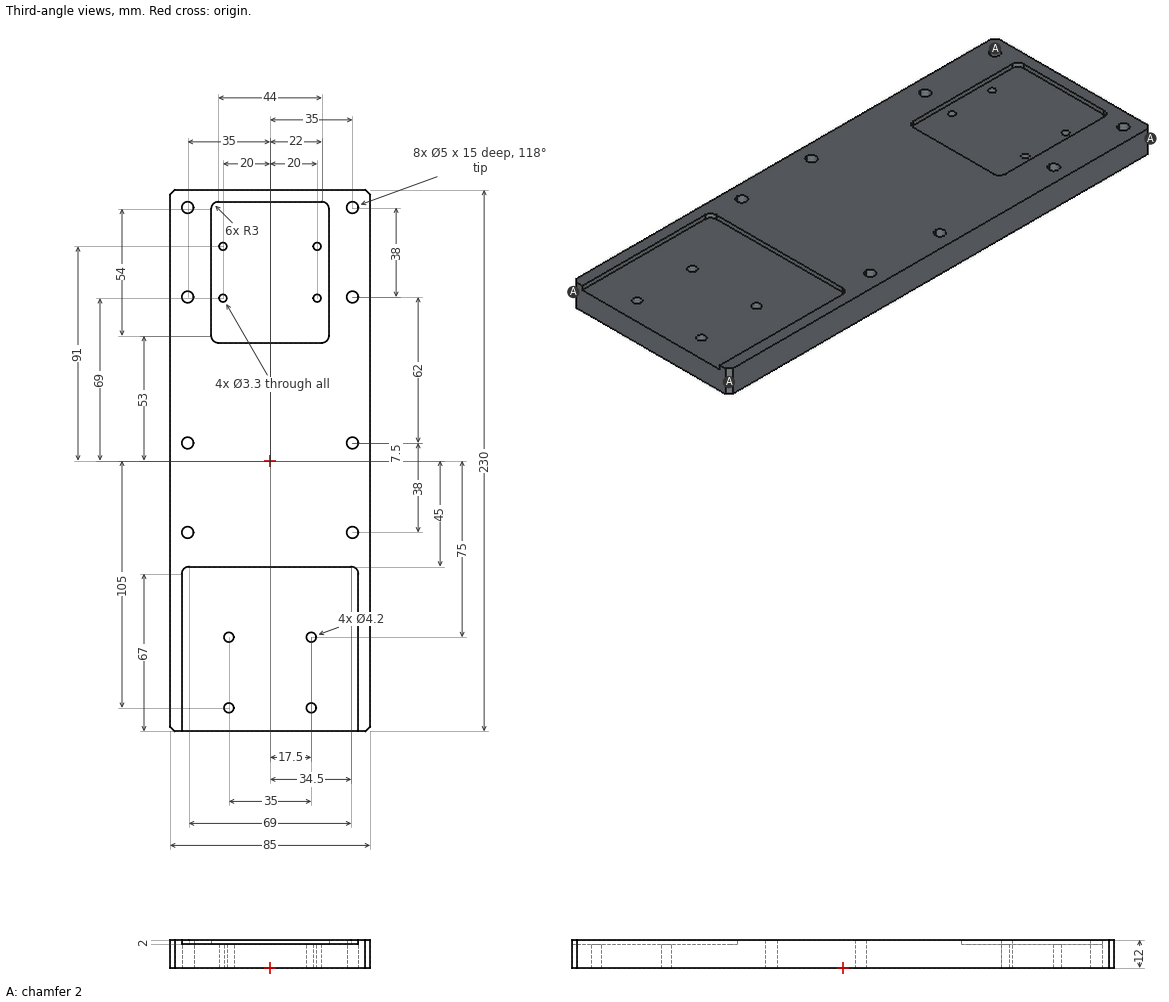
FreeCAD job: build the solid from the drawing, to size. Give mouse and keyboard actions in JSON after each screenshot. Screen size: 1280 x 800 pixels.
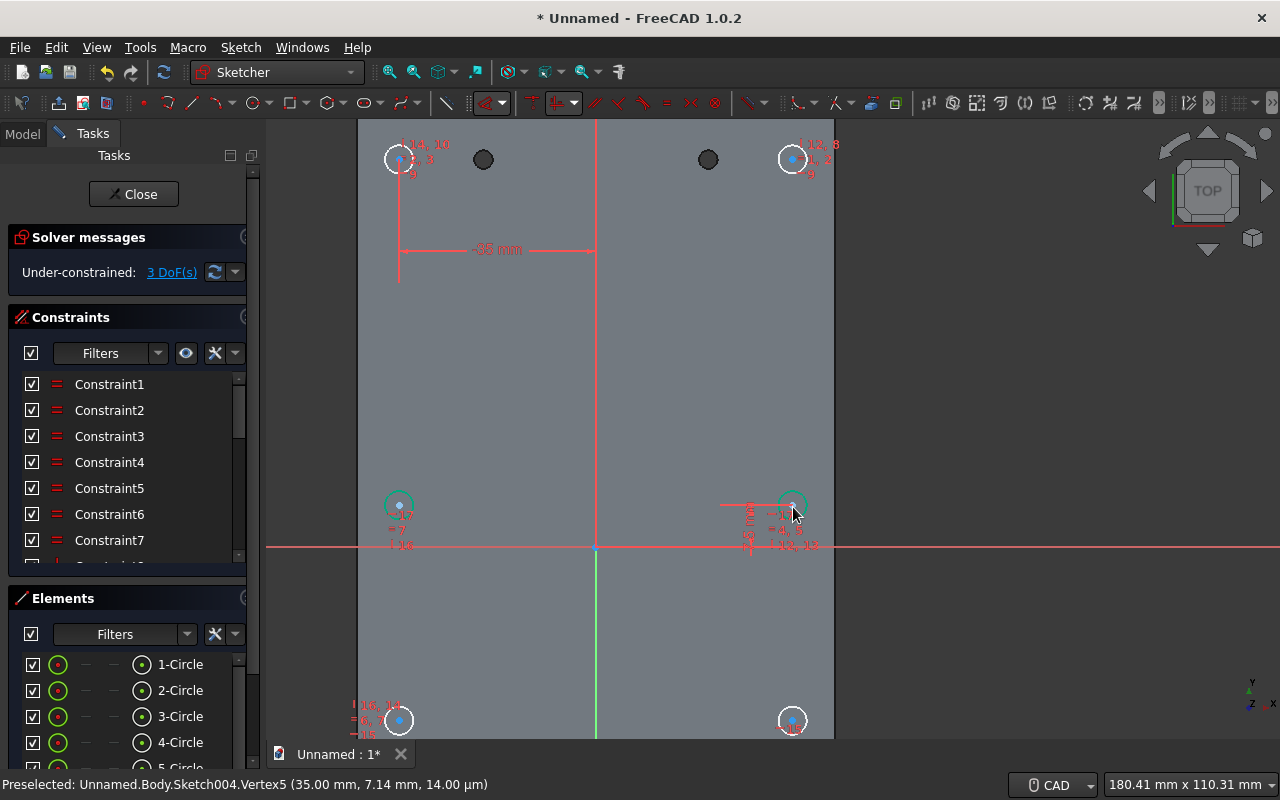
{"action": "scroll", "coordinate": [793, 509], "scroll_direction": "down", "scroll_amount": 4}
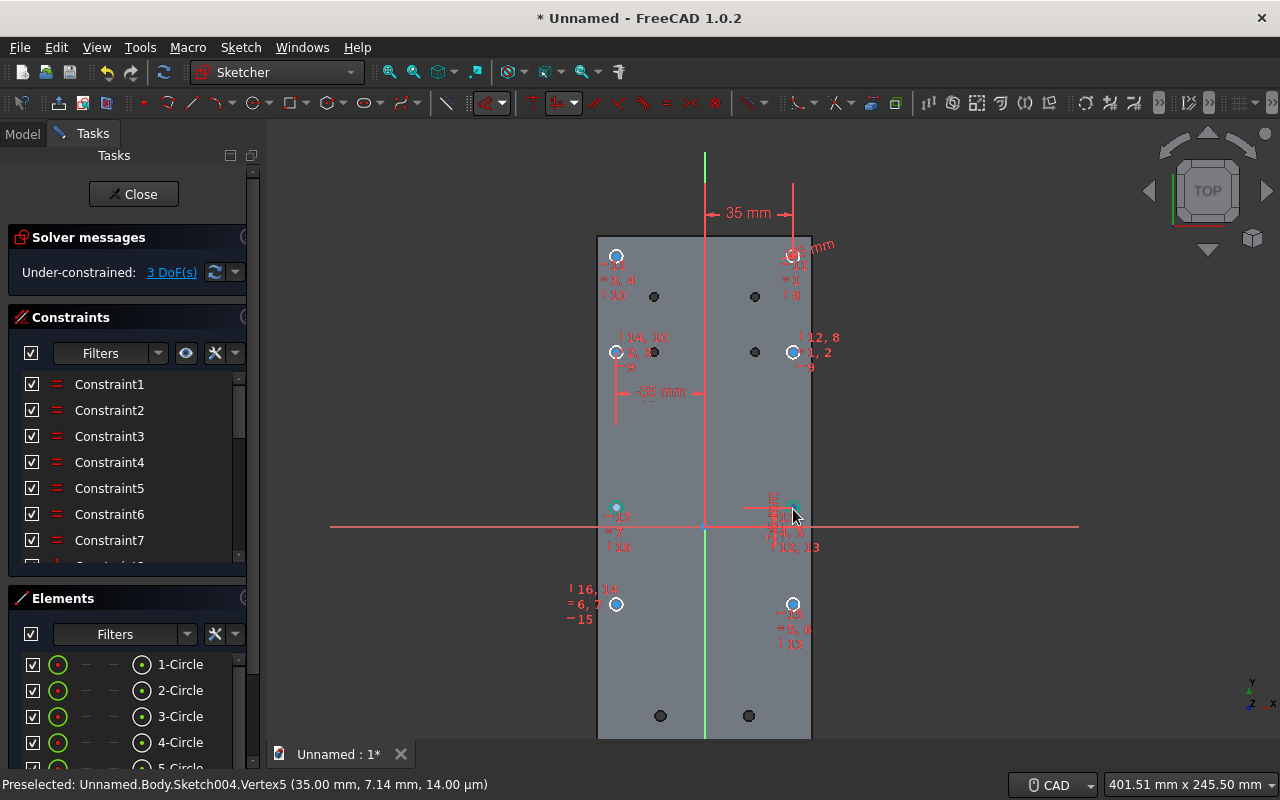
{"action": "left_click", "coordinate": [793, 256]}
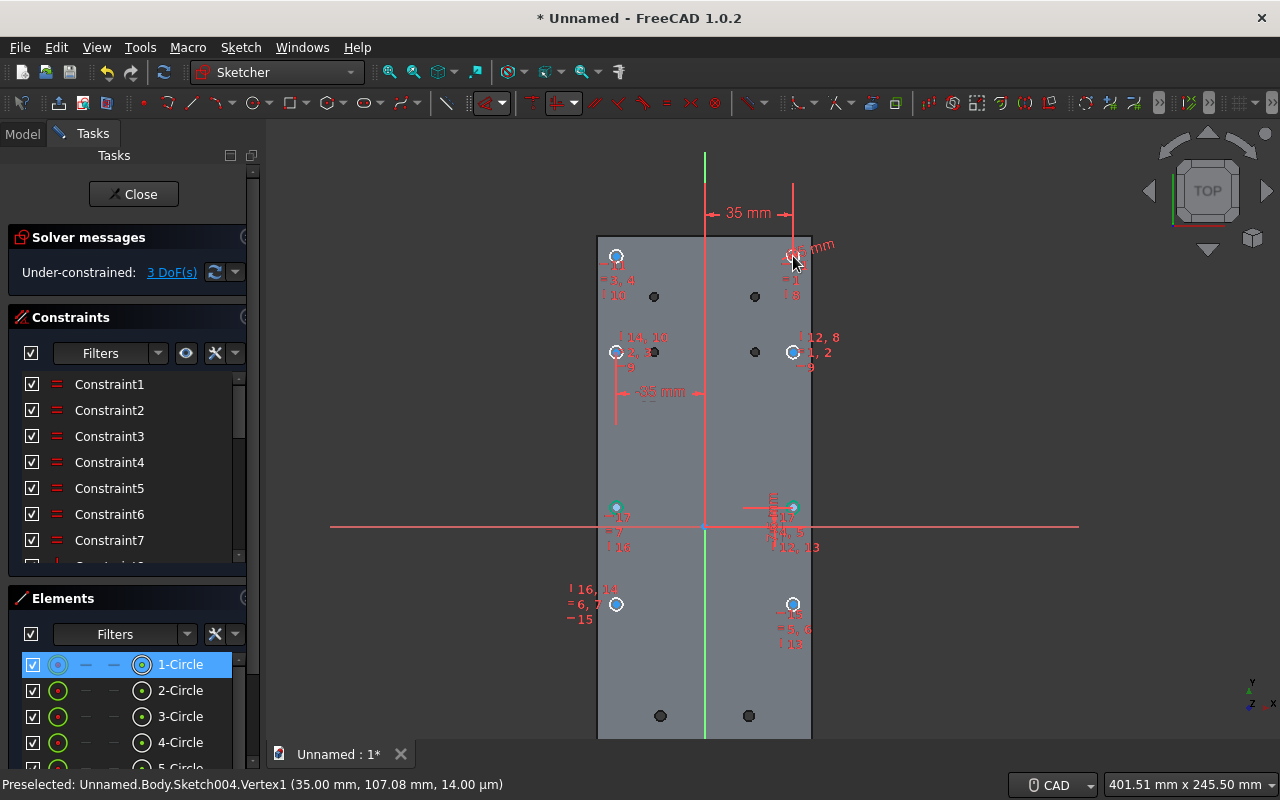
{"action": "left_click", "coordinate": [793, 352]}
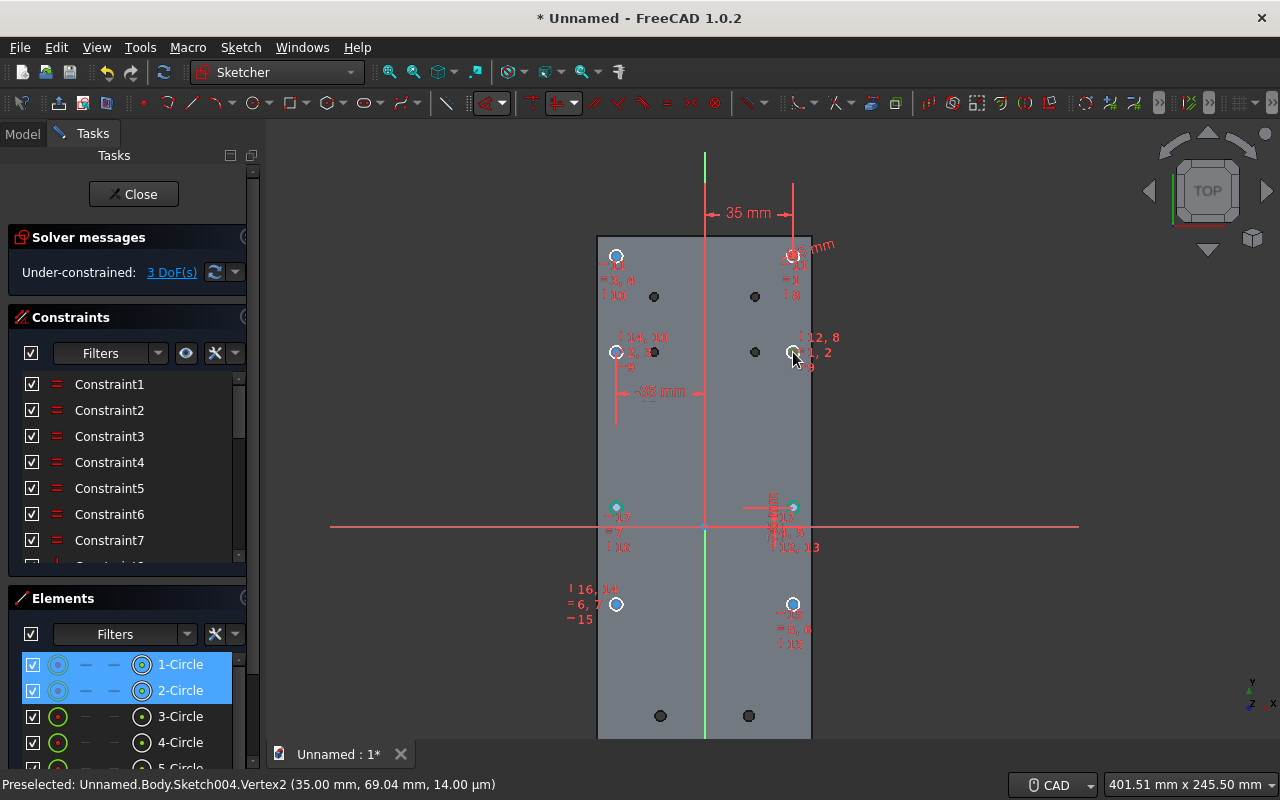
{"action": "left_click", "coordinate": [504, 104]}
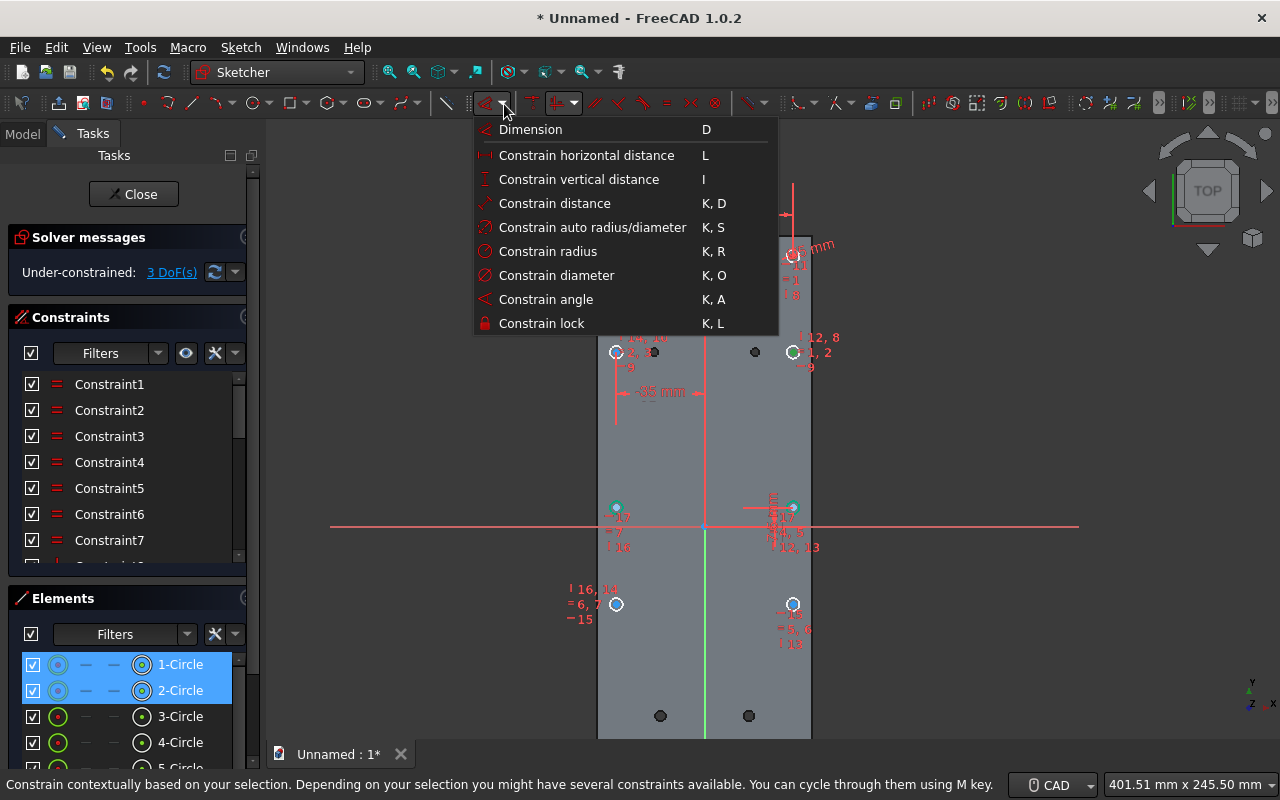
{"action": "left_click", "coordinate": [626, 179]}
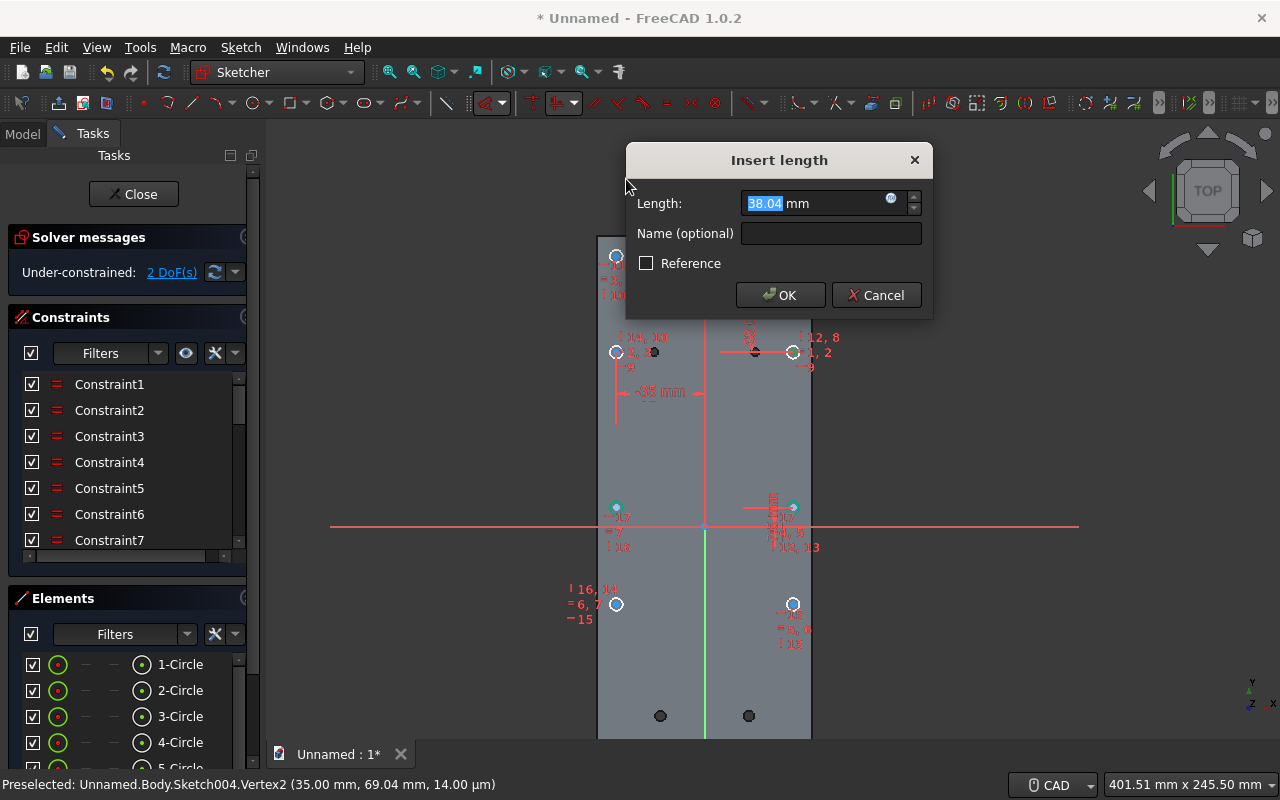
{"action": "type", "text": "38"}
{"action": "key", "text": "Return"}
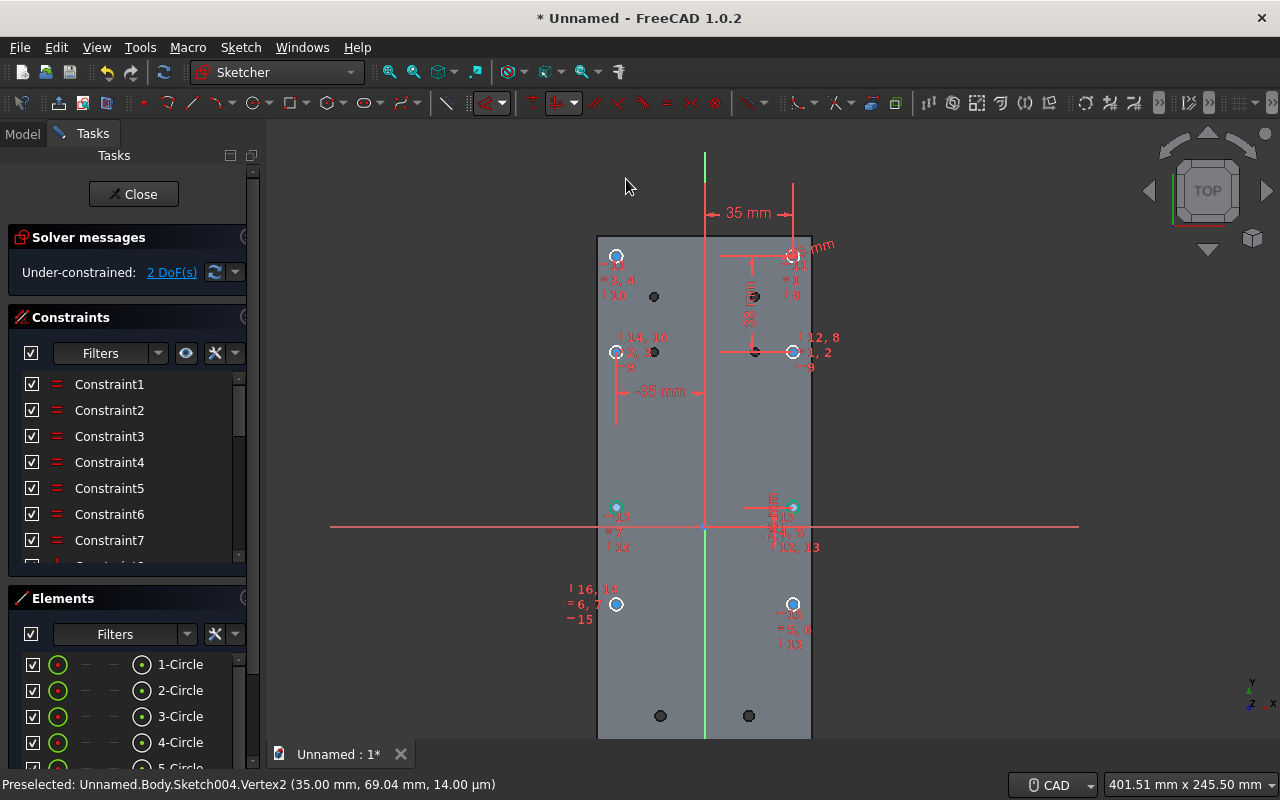
{"action": "left_click", "coordinate": [793, 352]}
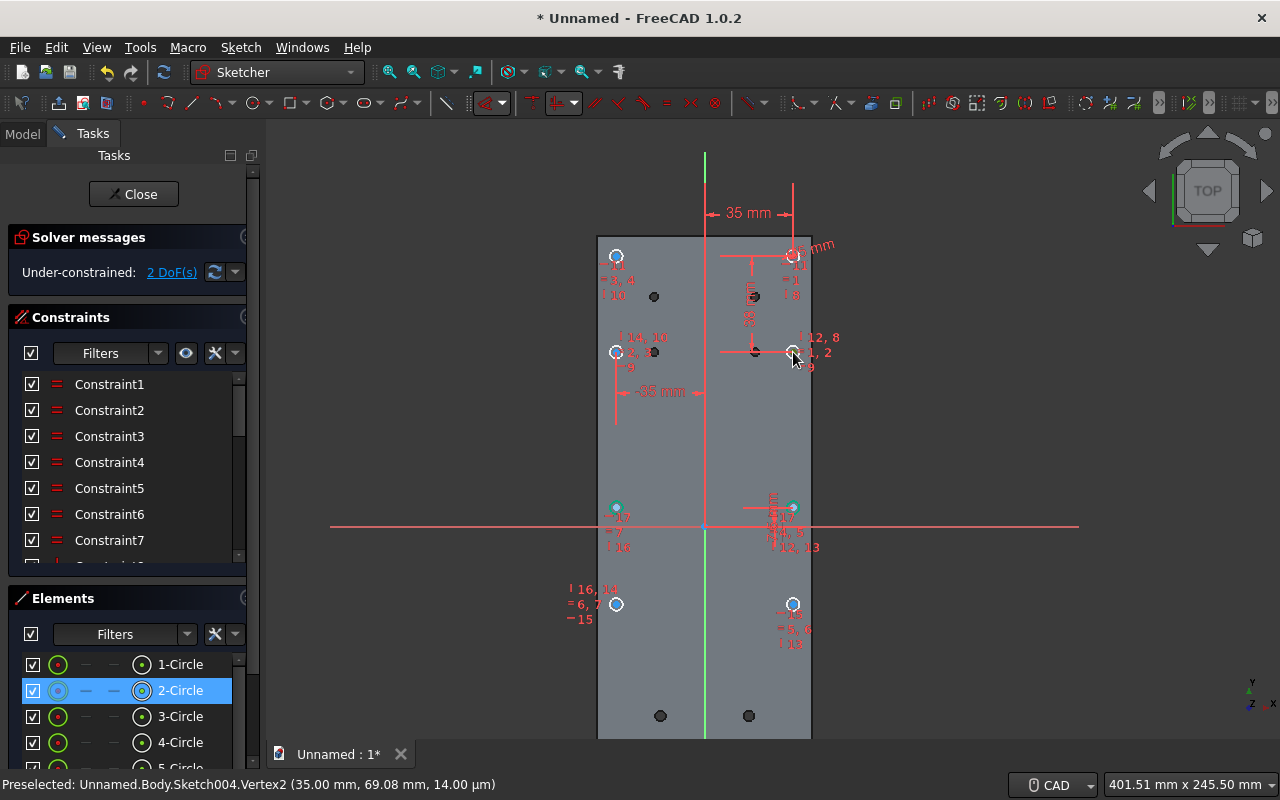
{"action": "left_click", "coordinate": [793, 508]}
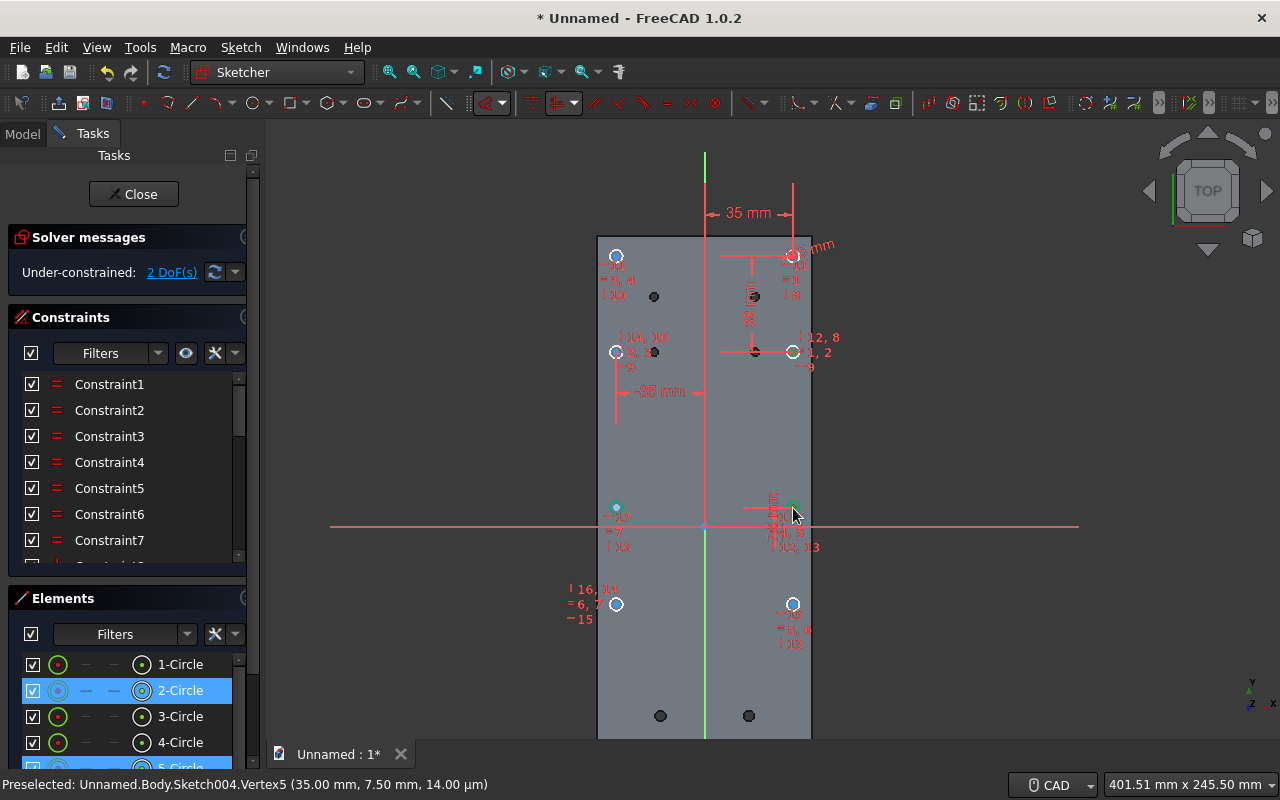
{"action": "key", "text": "i"}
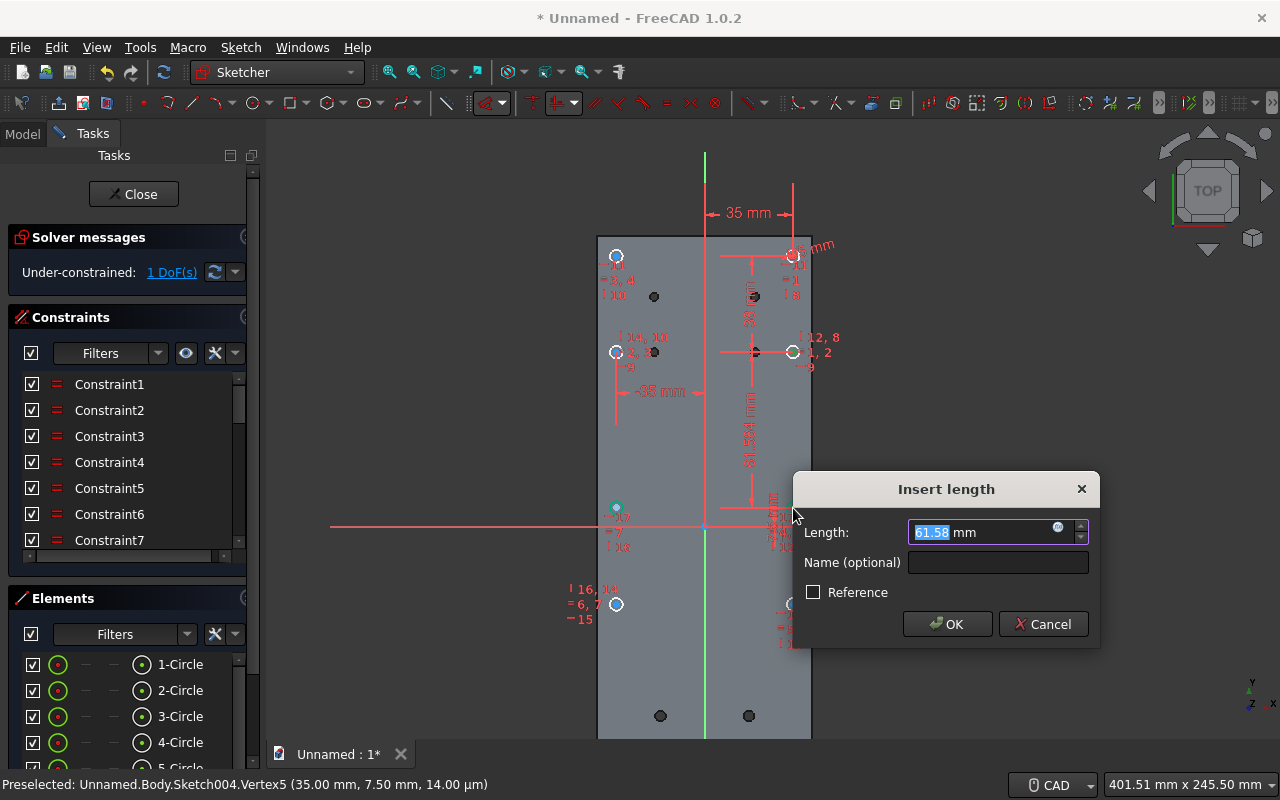
{"action": "type", "text": "62"}
{"action": "key", "text": "Return"}